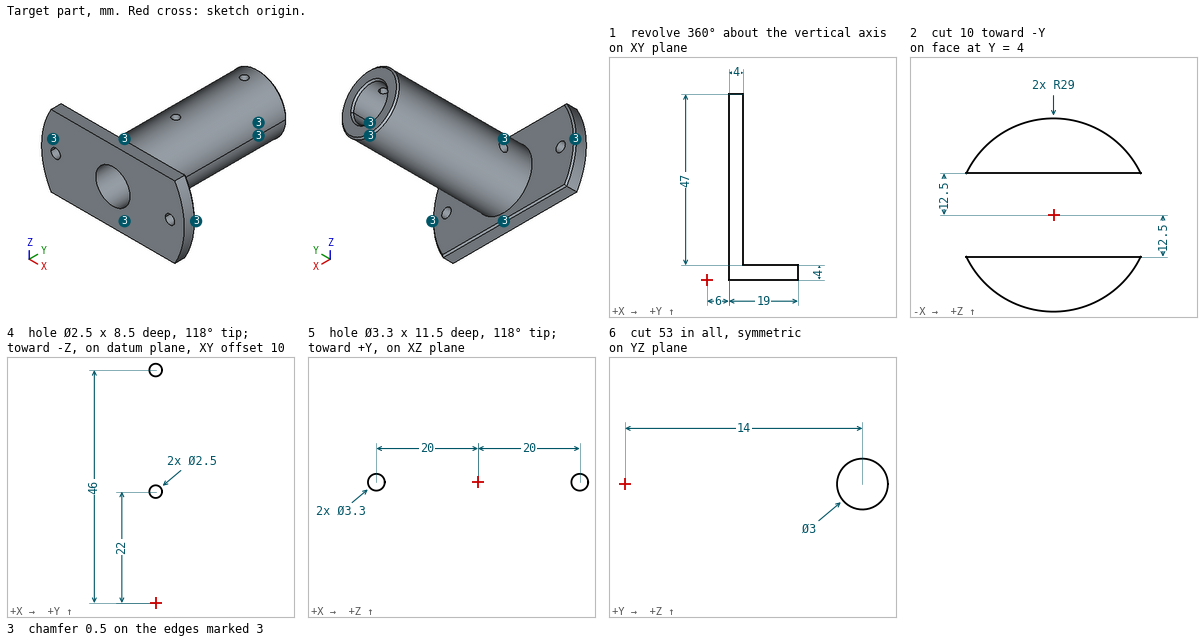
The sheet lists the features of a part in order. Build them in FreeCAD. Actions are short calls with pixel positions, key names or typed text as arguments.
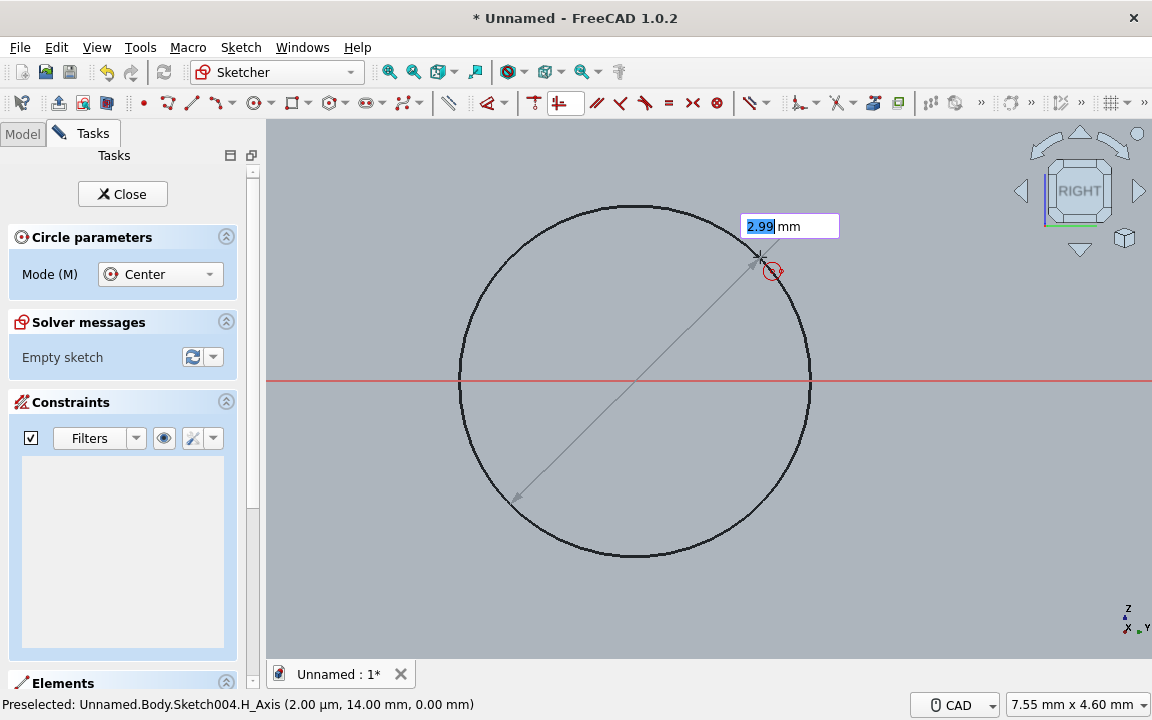
text(3)
key(Return)
key(Escape)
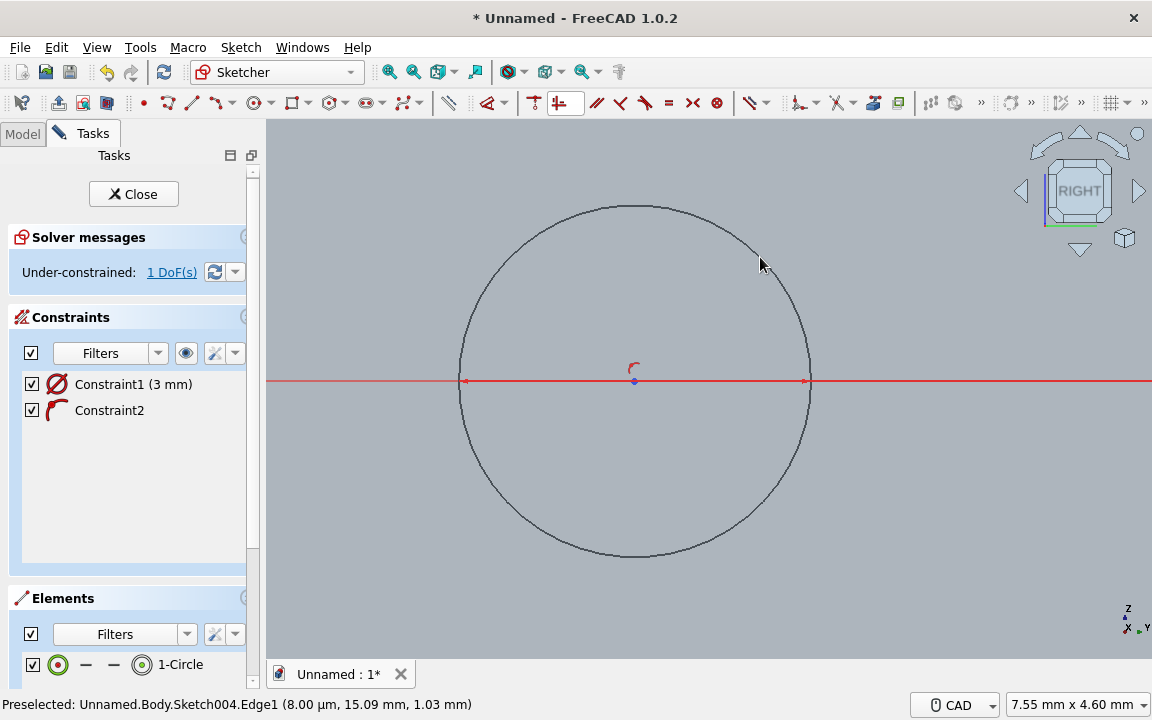
click(488, 104)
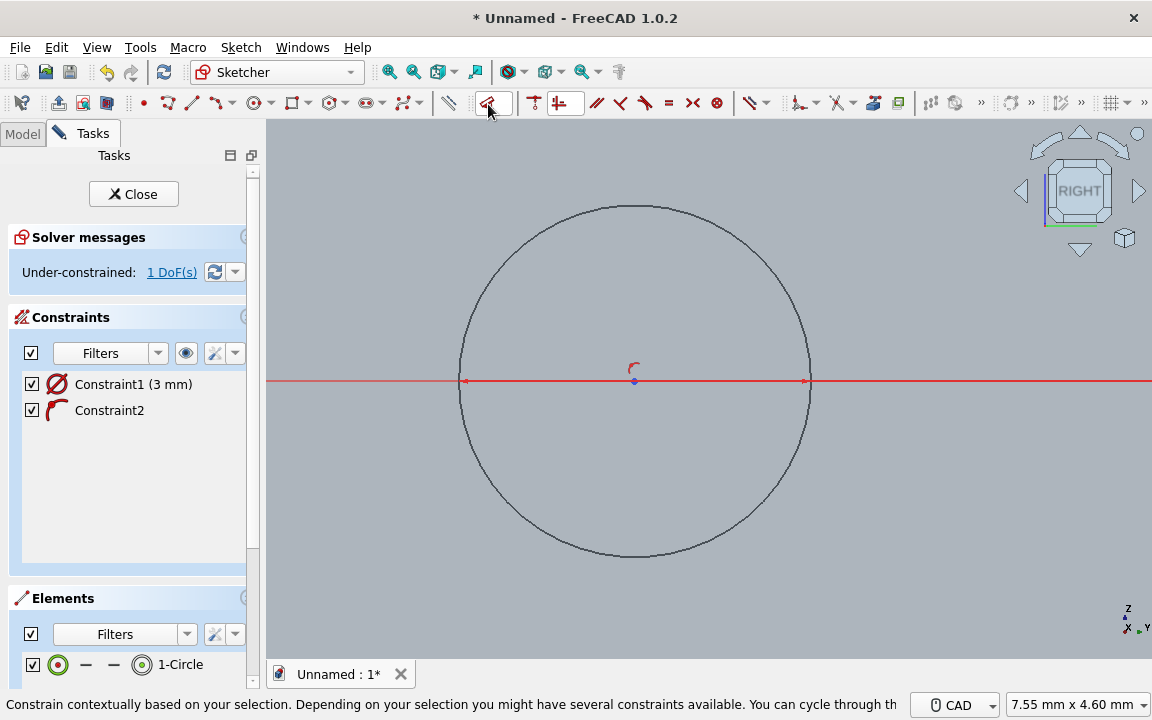
click(635, 381)
click(386, 415)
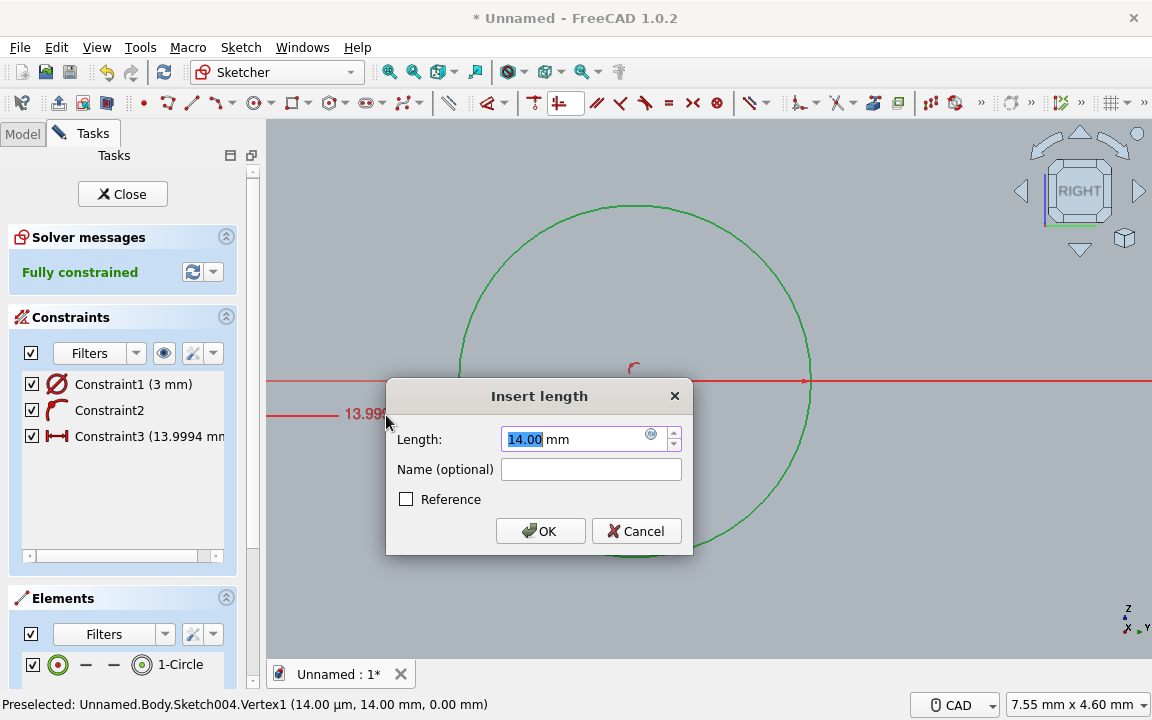
text(14)
key(Return)
key(Escape)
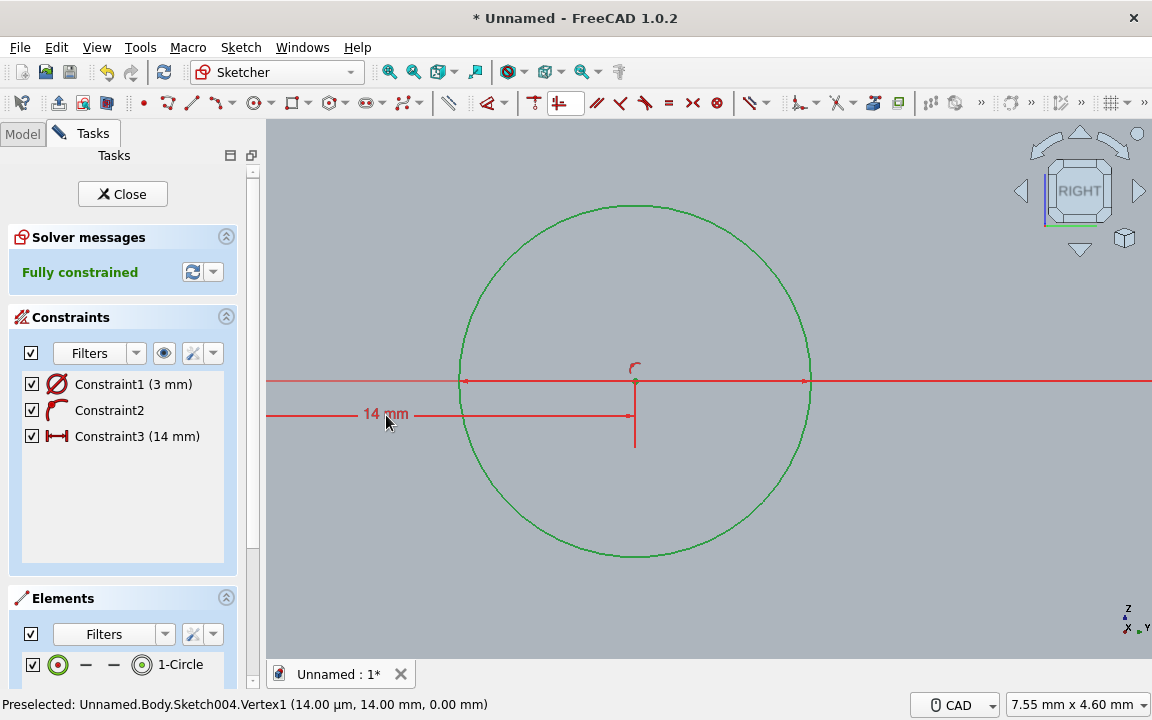
click(123, 194)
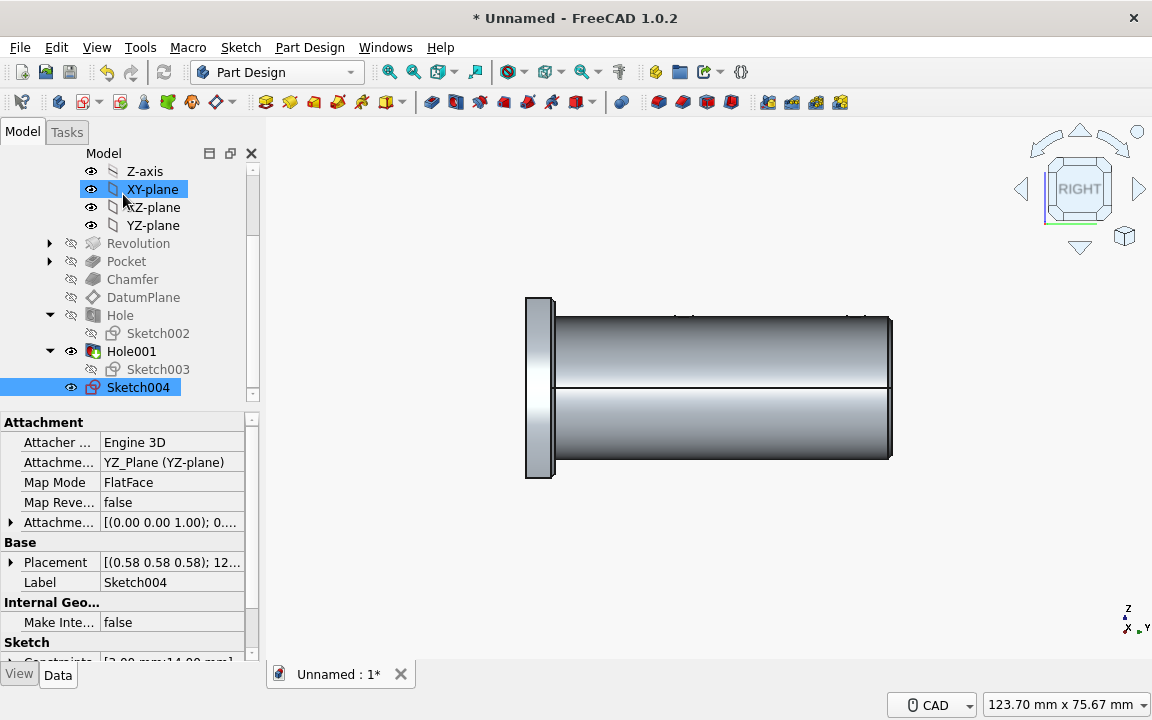
click(432, 102)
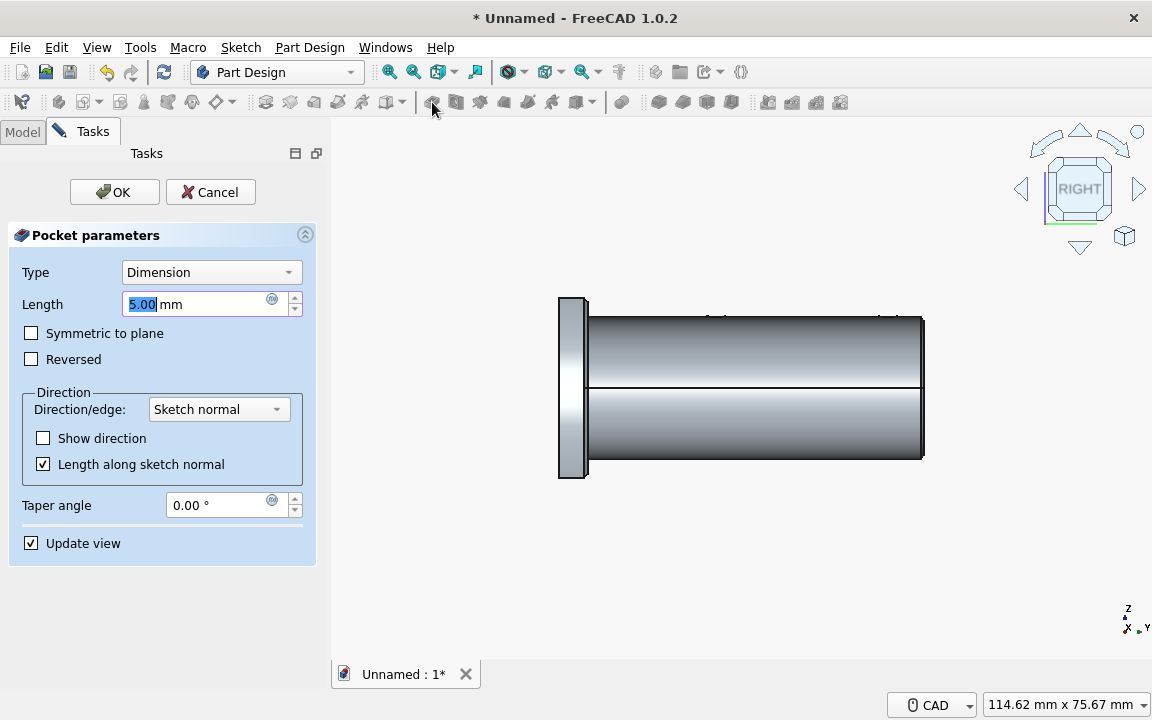
text(53)
key(Tab)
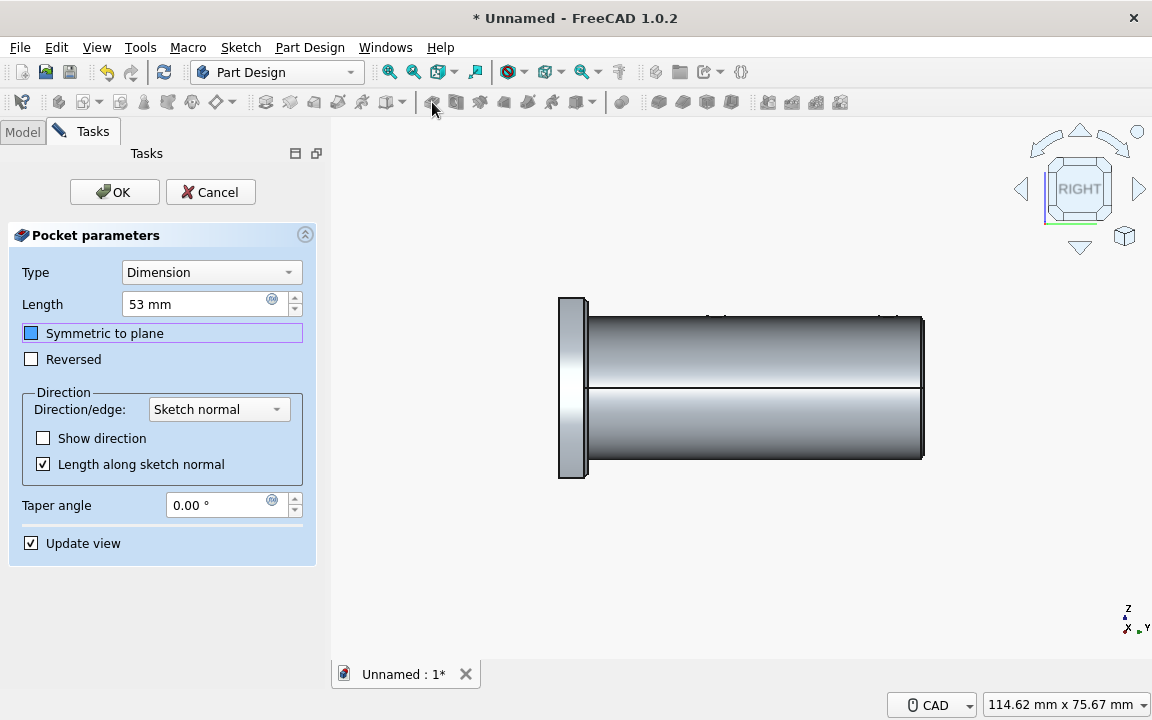
click(30, 333)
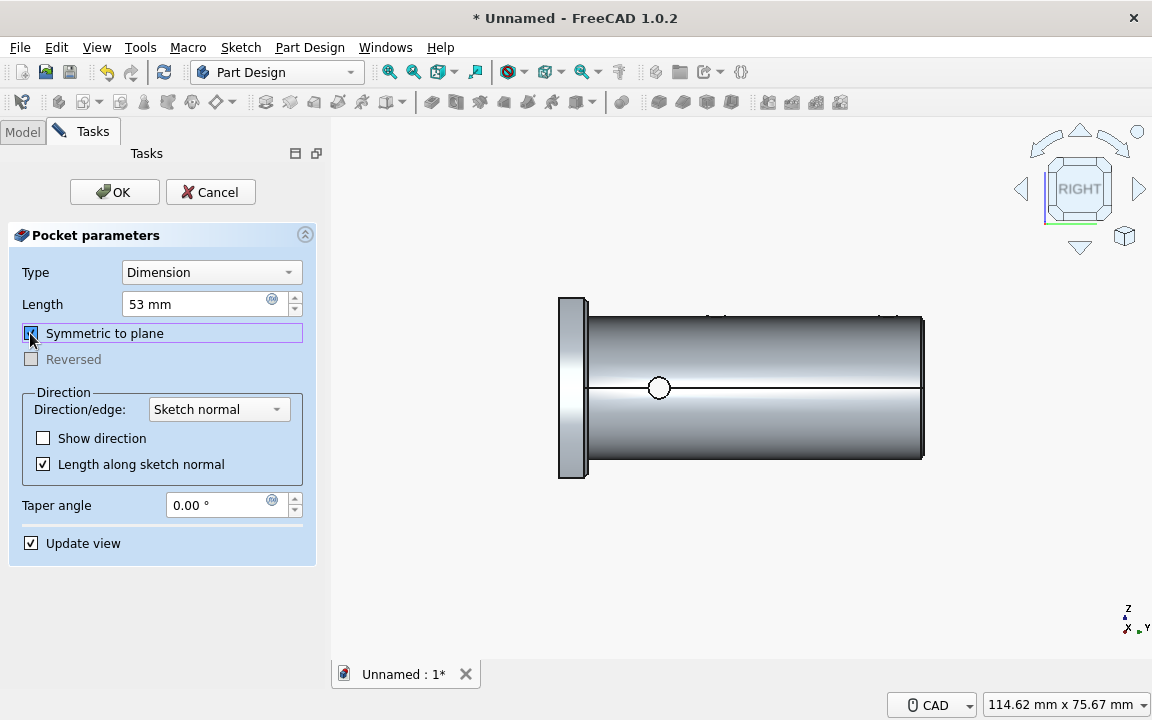
click(115, 192)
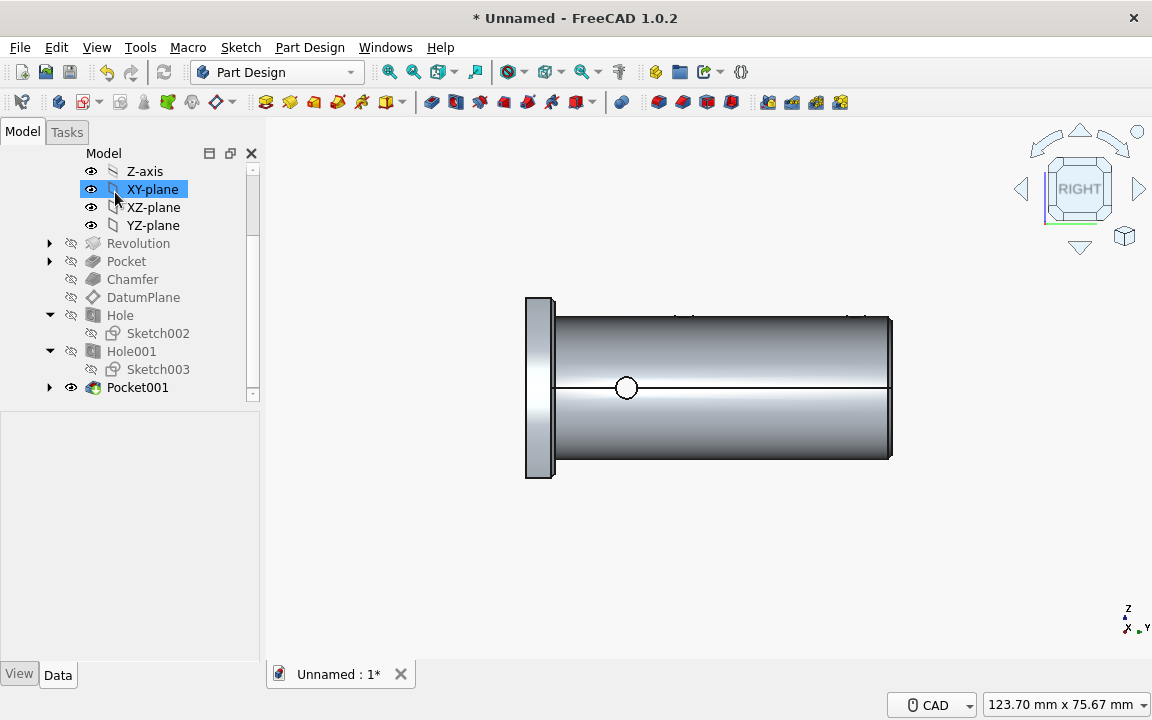
key(0)